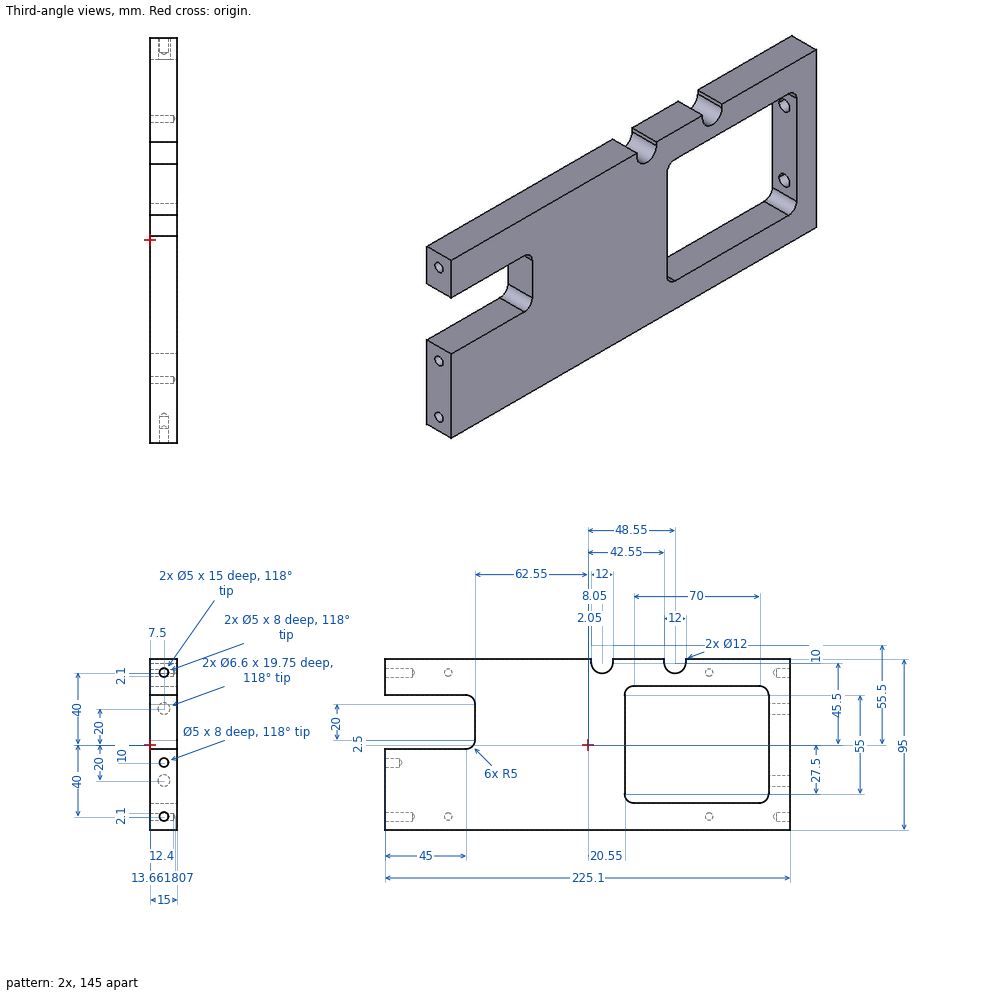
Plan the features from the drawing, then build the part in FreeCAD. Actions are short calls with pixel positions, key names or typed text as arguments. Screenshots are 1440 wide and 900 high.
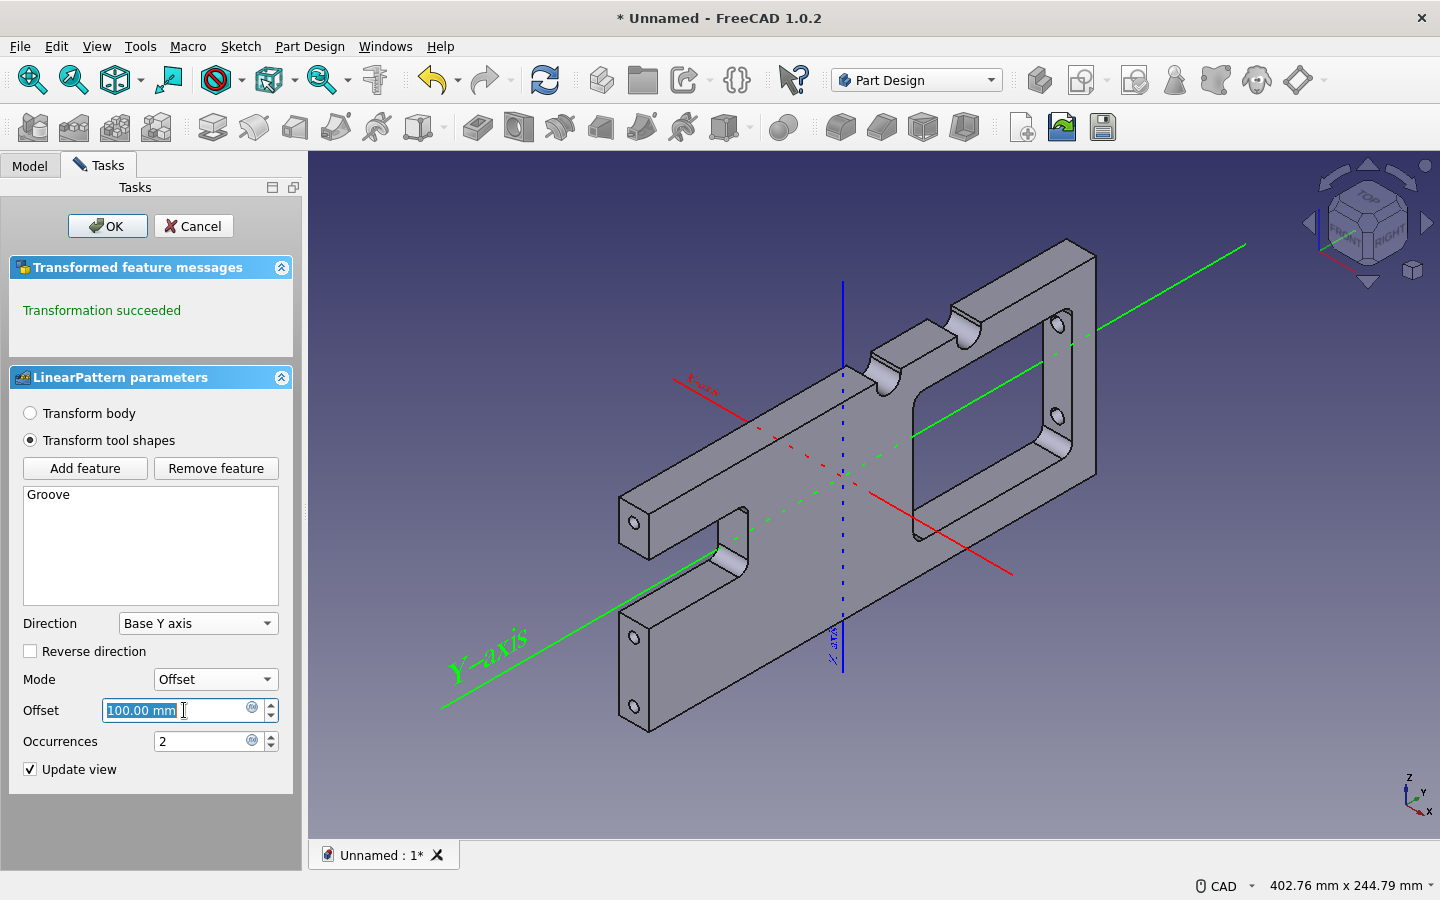
text(145)
key(Tab)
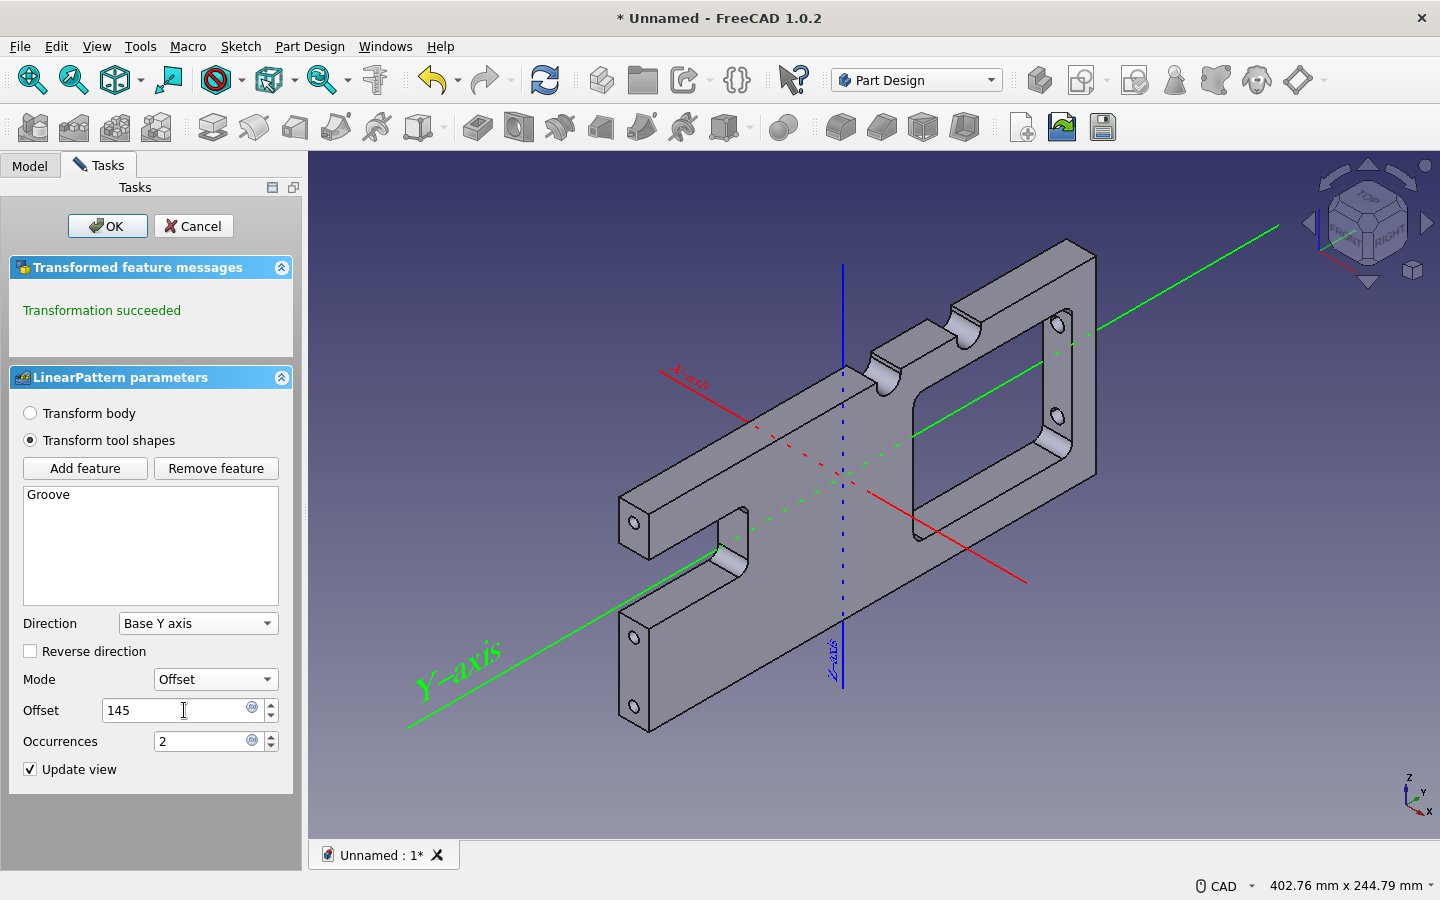
triple_click(210, 742)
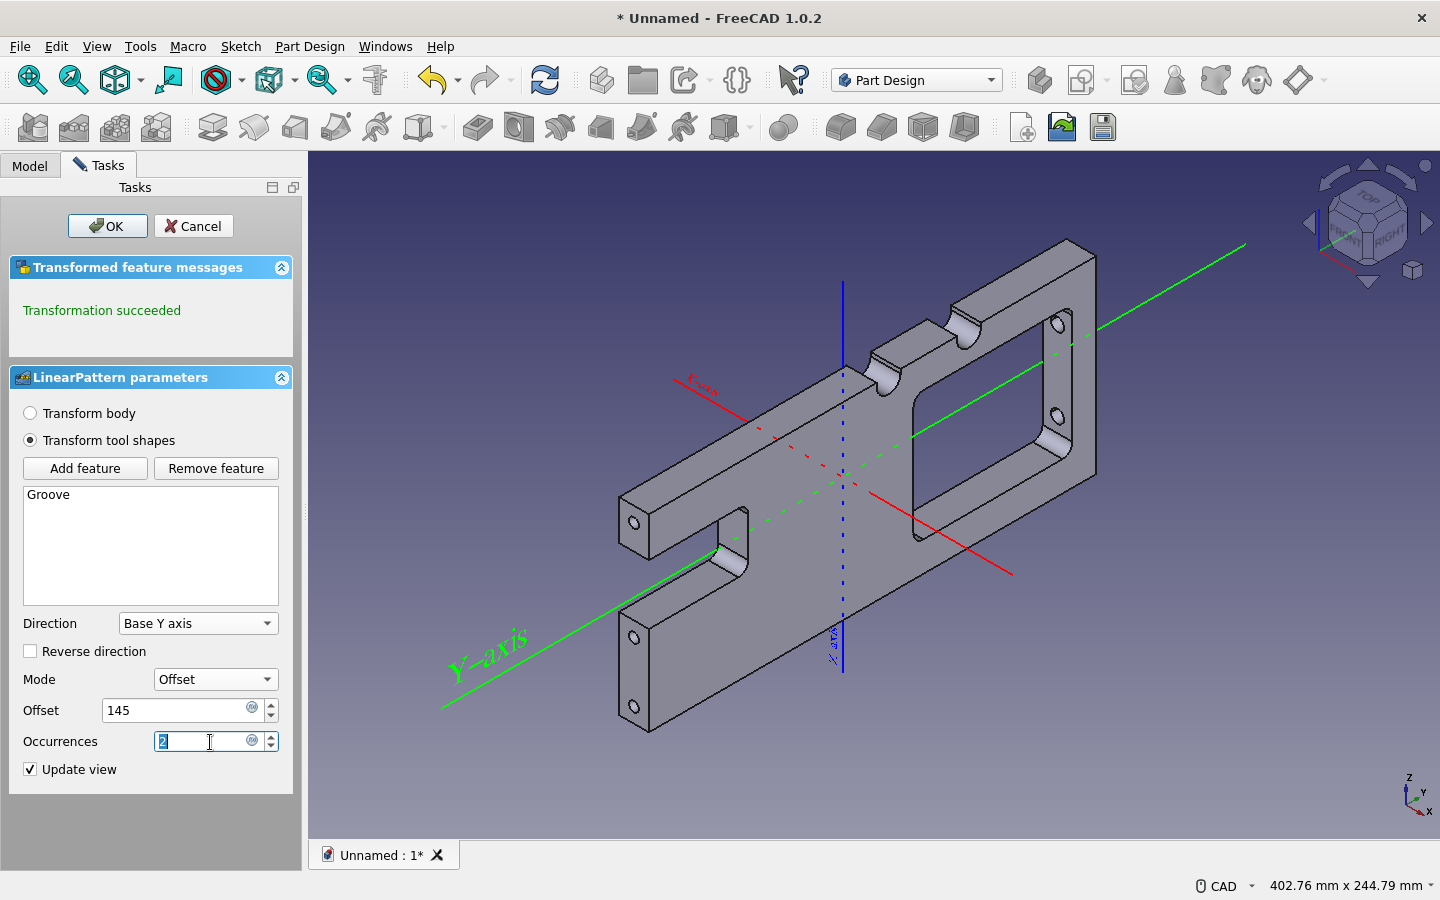
text(2)
key(Tab)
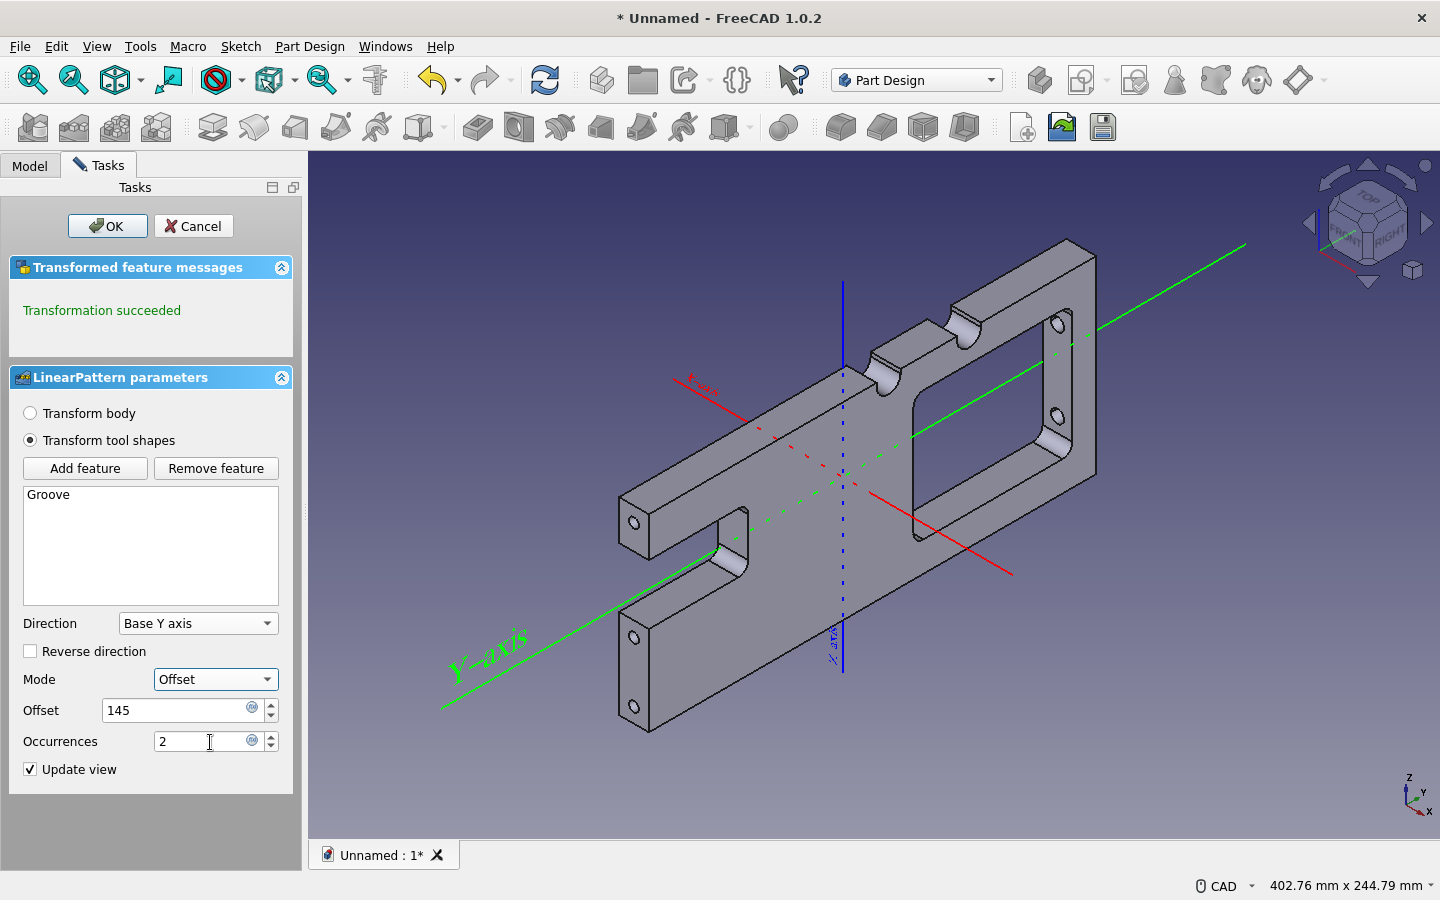
click(108, 226)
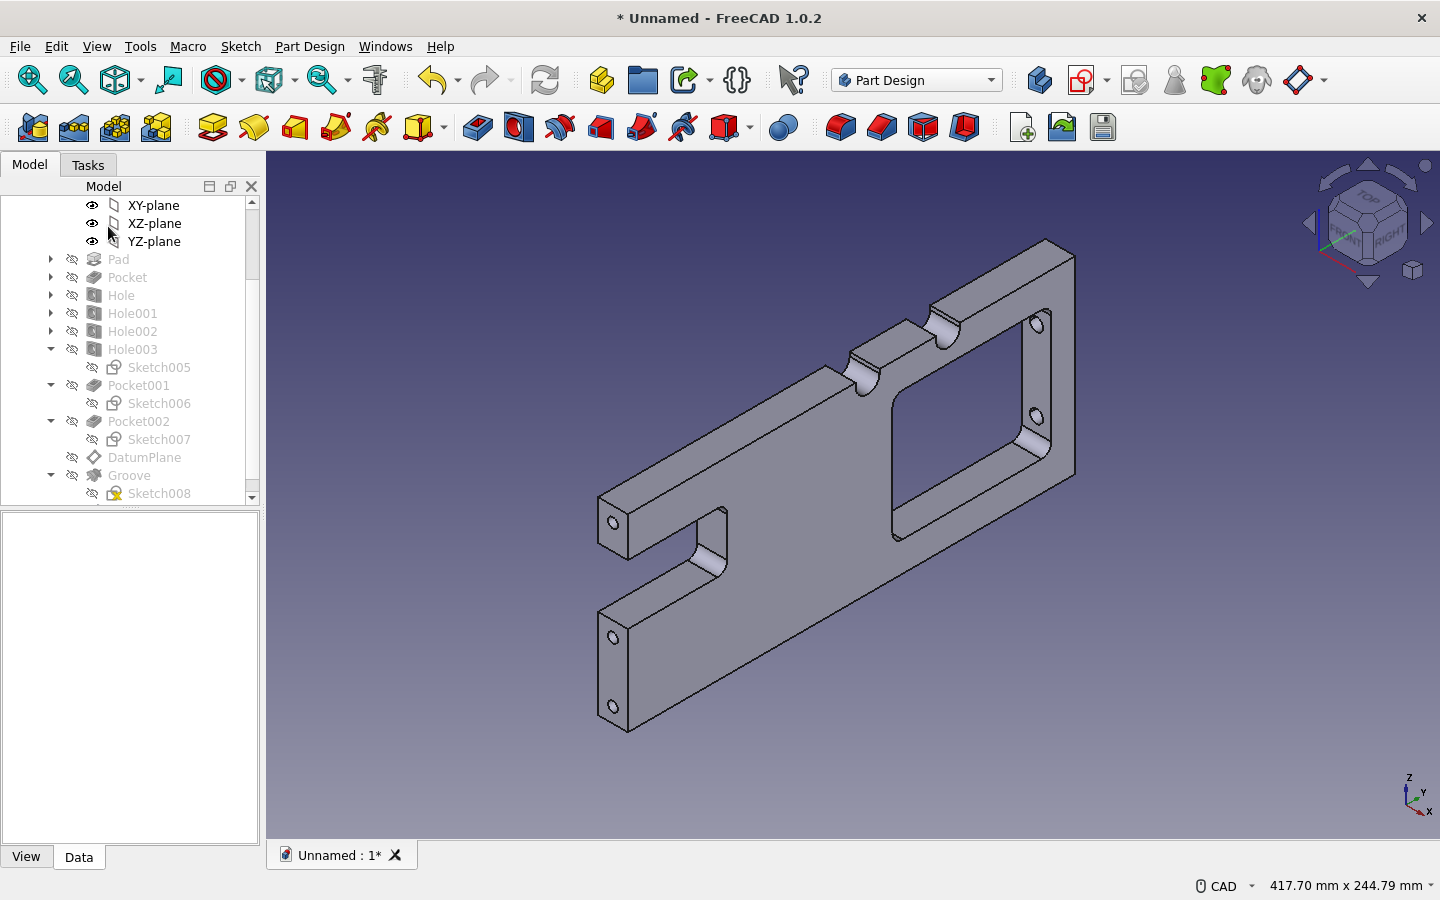
click(117, 475)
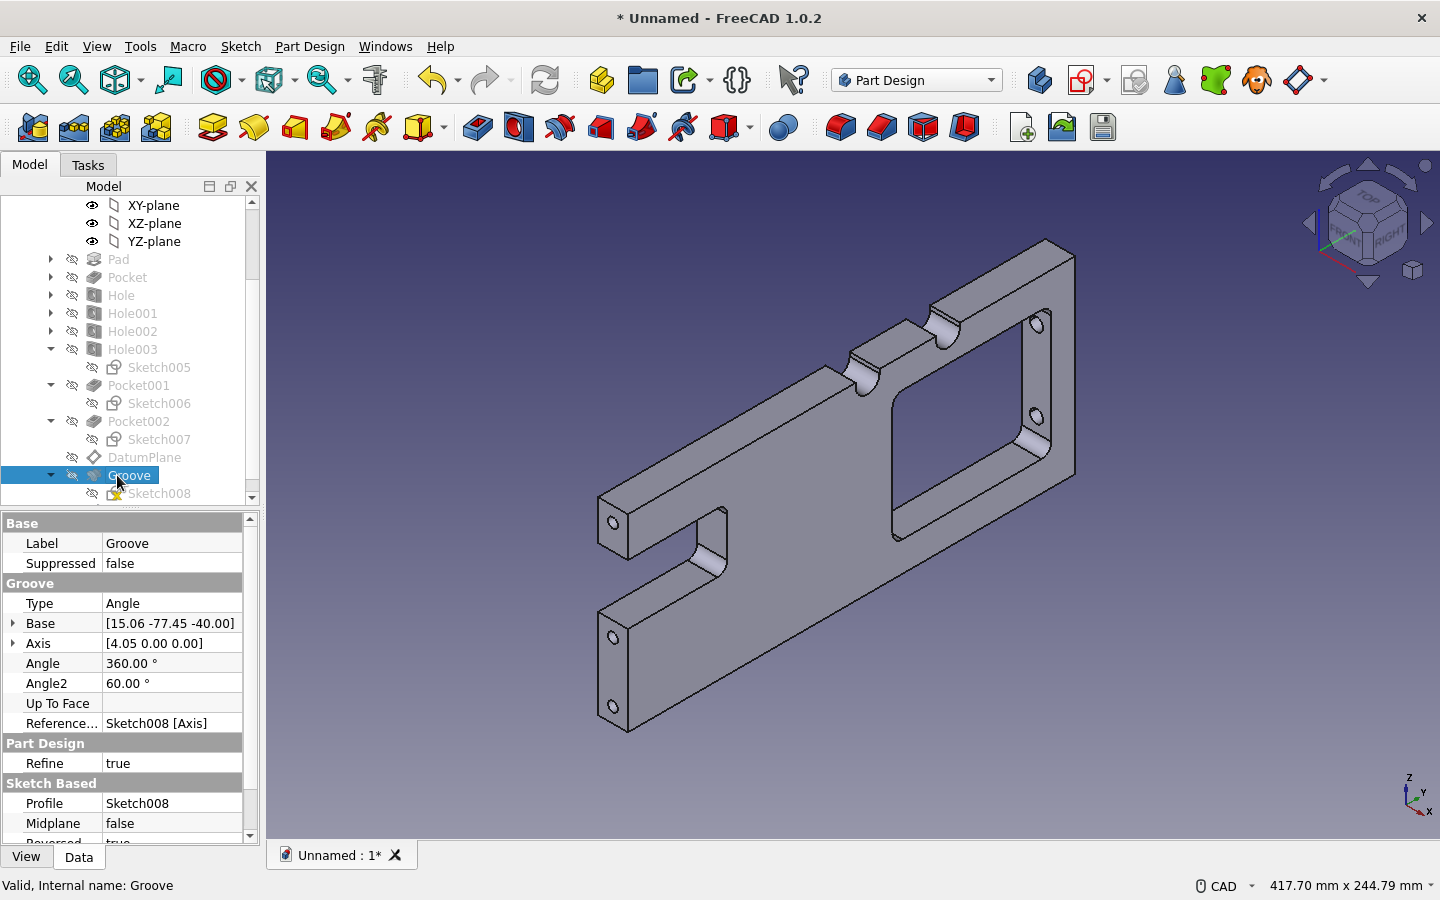
click(33, 128)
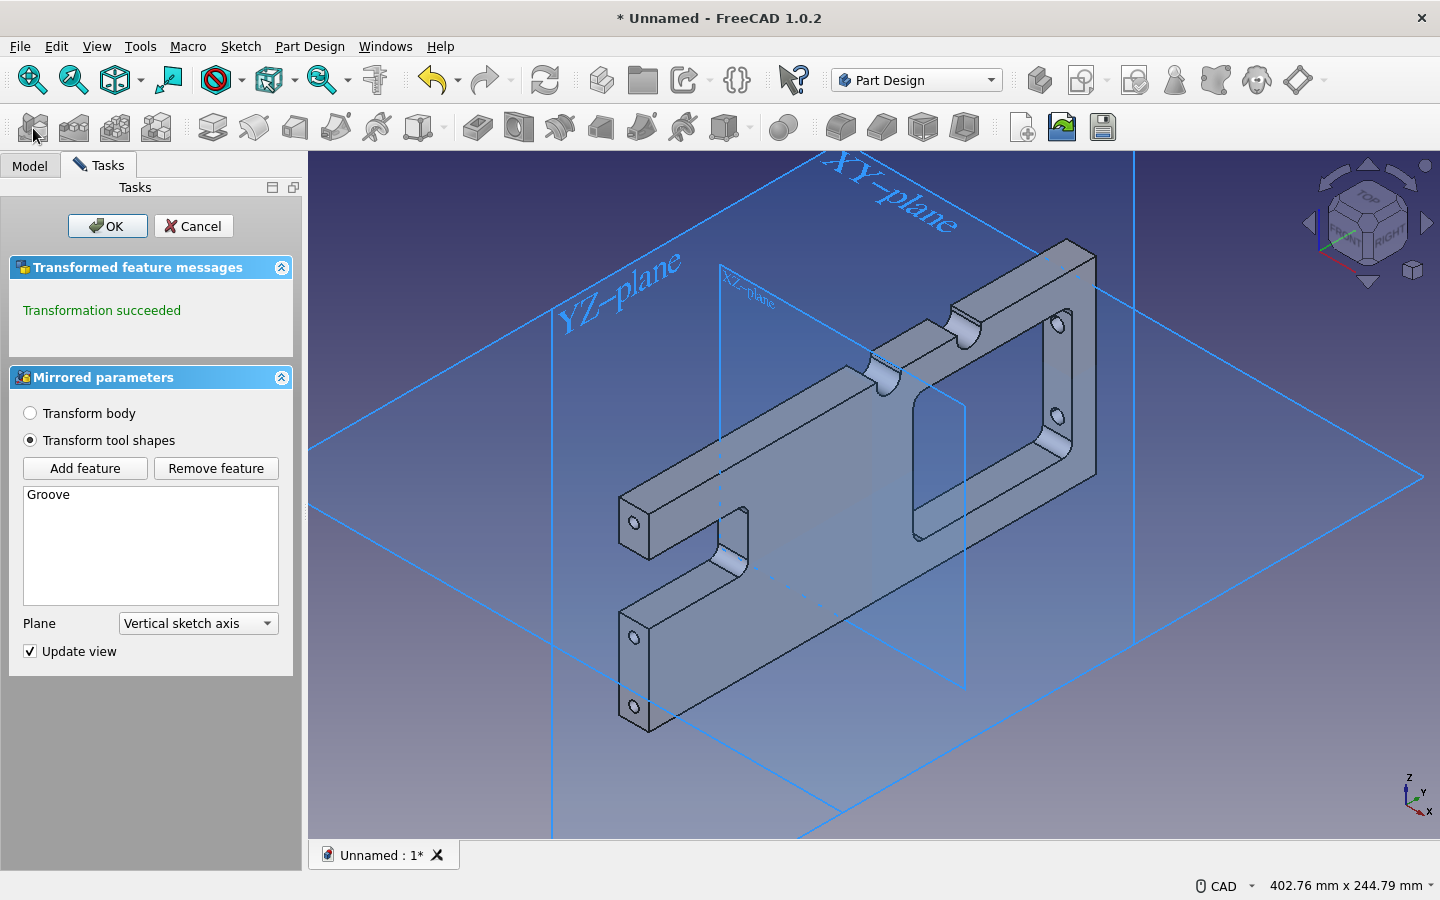
click(199, 624)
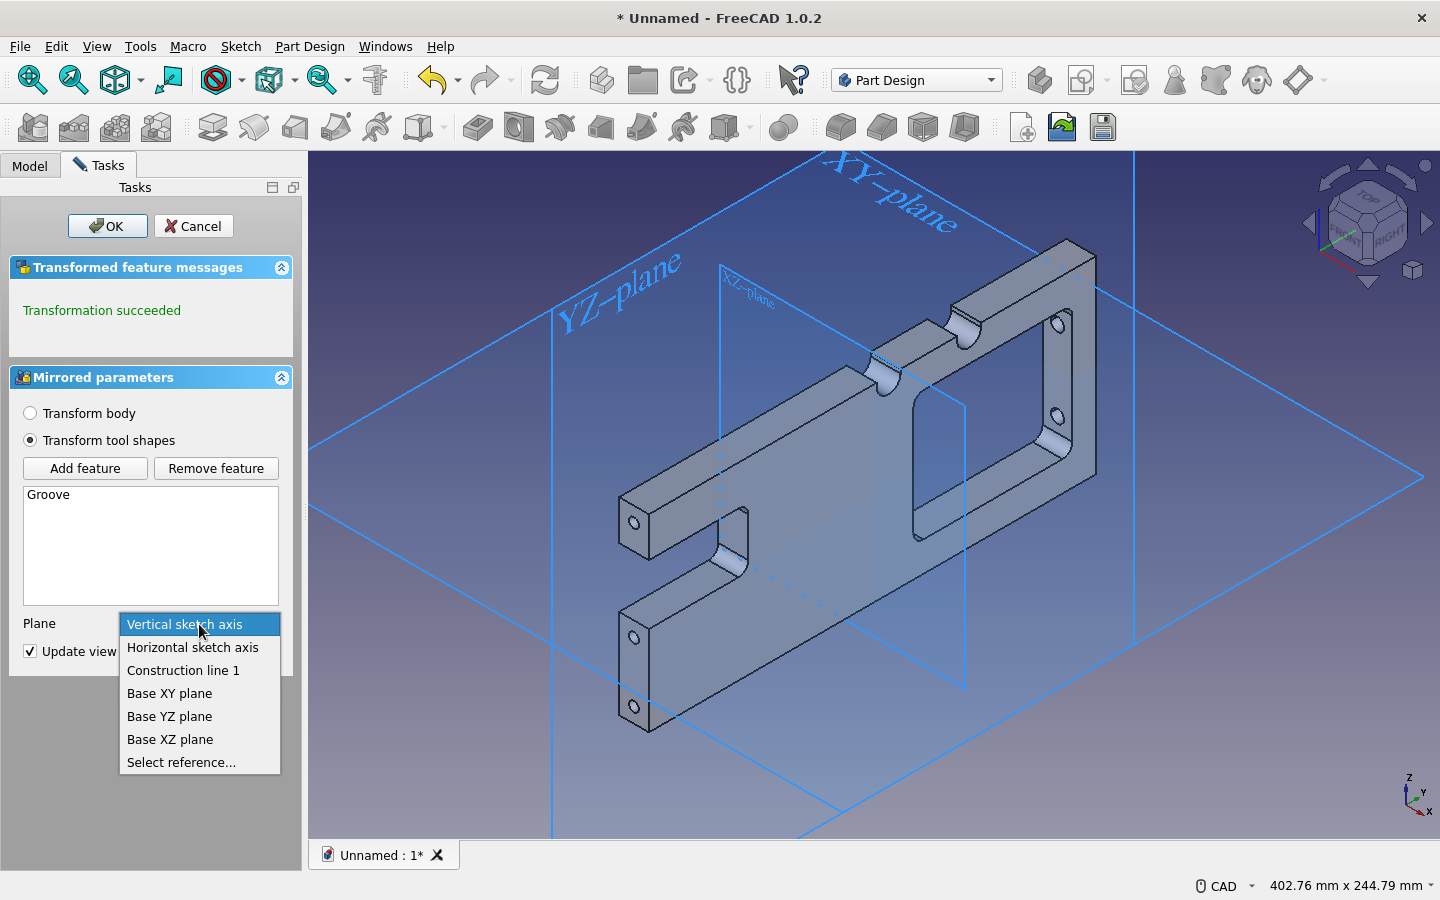
click(198, 694)